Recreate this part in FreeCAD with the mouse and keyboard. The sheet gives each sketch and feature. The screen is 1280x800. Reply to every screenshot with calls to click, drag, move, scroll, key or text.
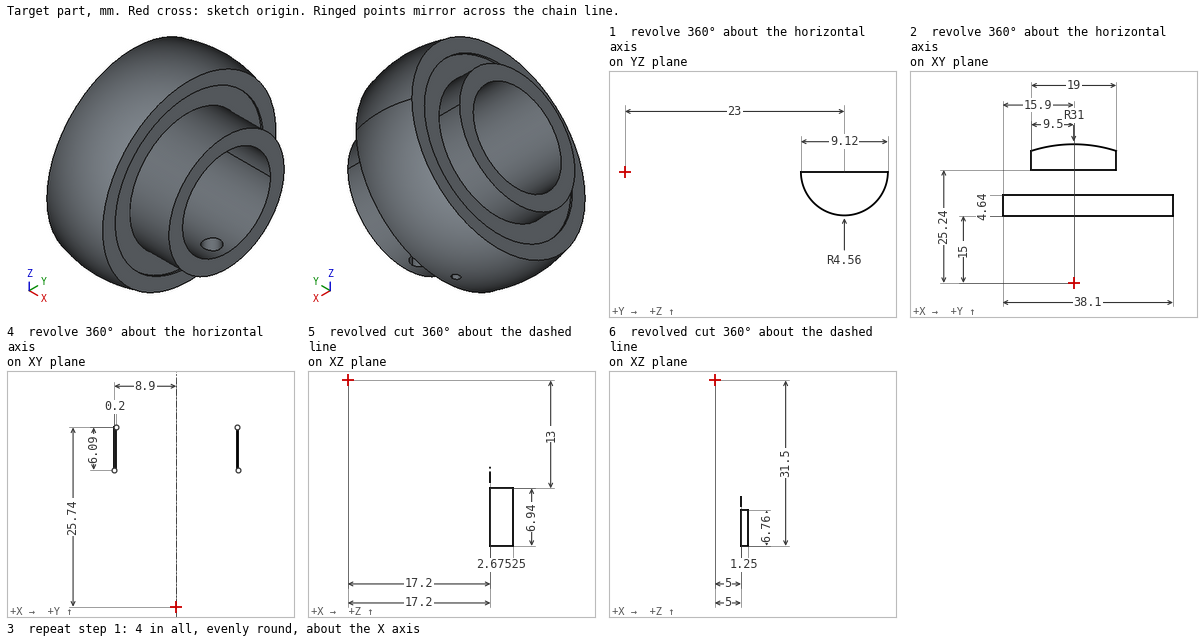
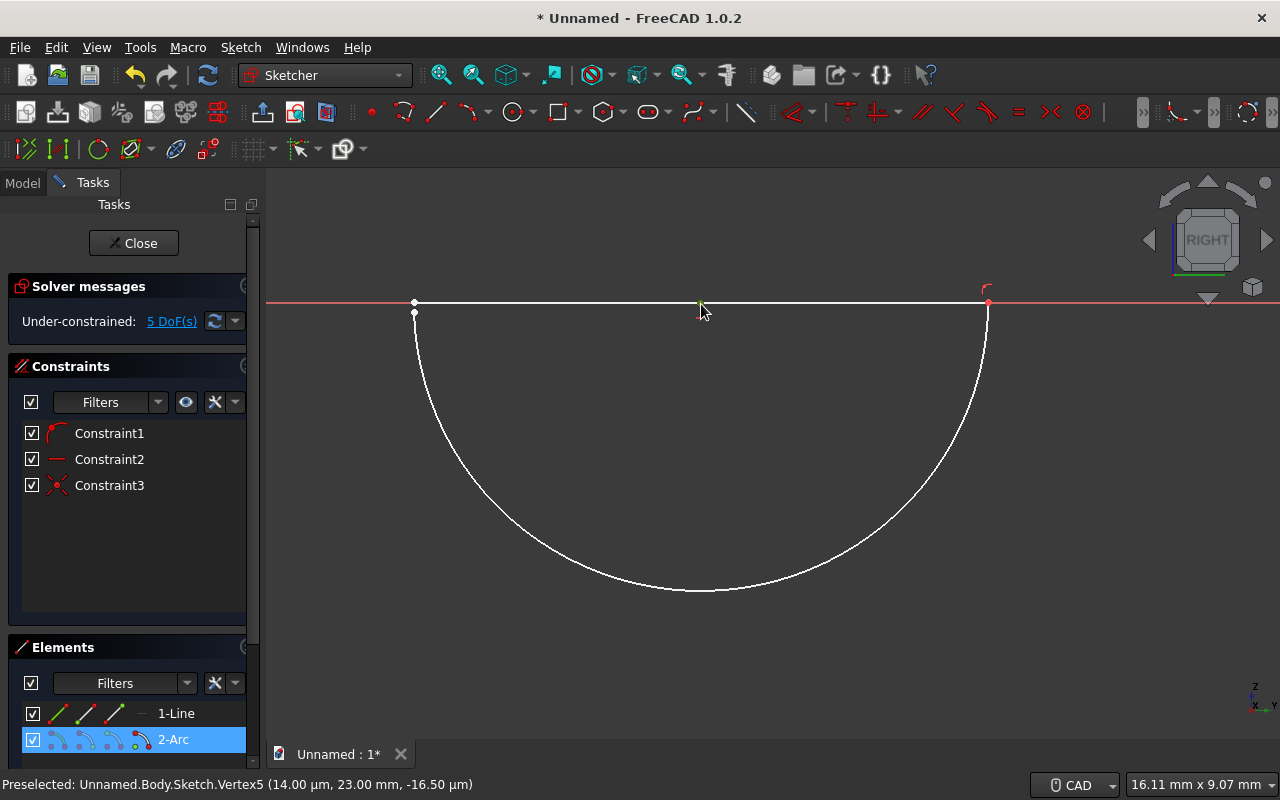
click(353, 303)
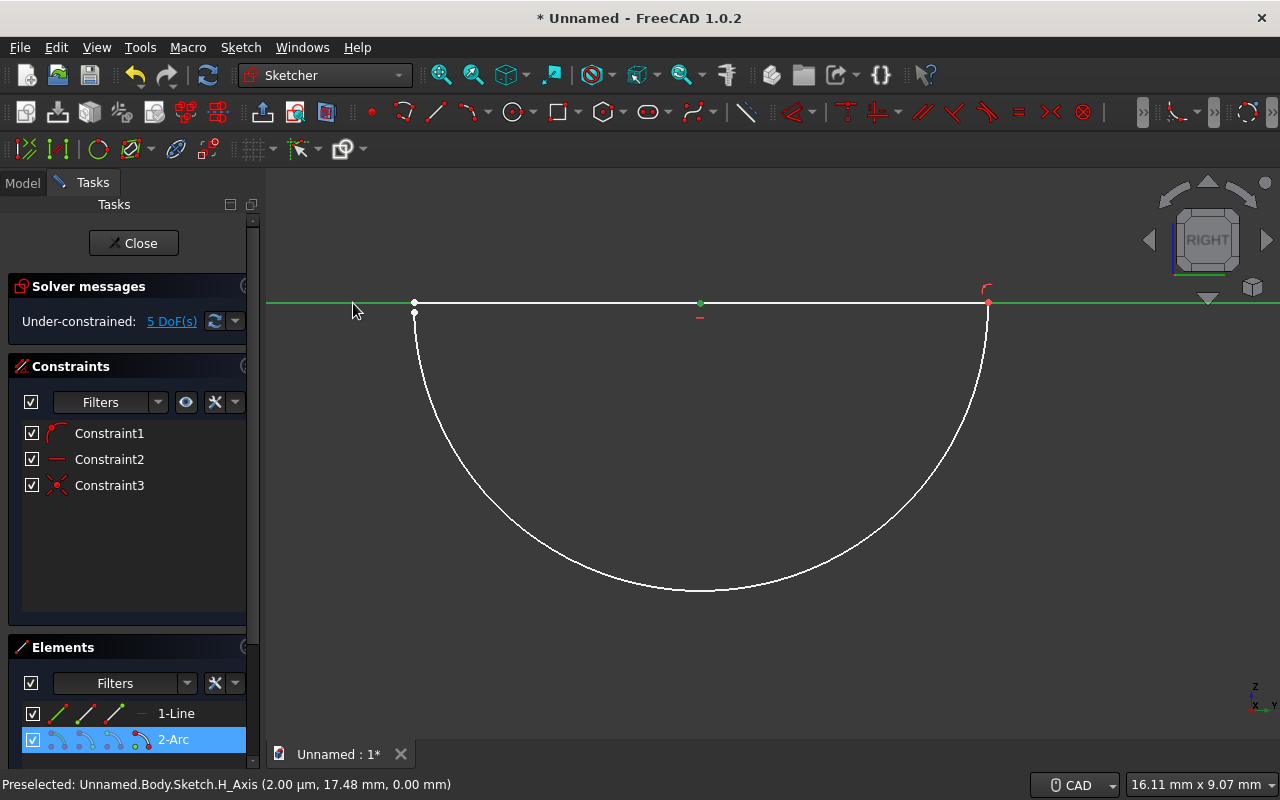
click(846, 112)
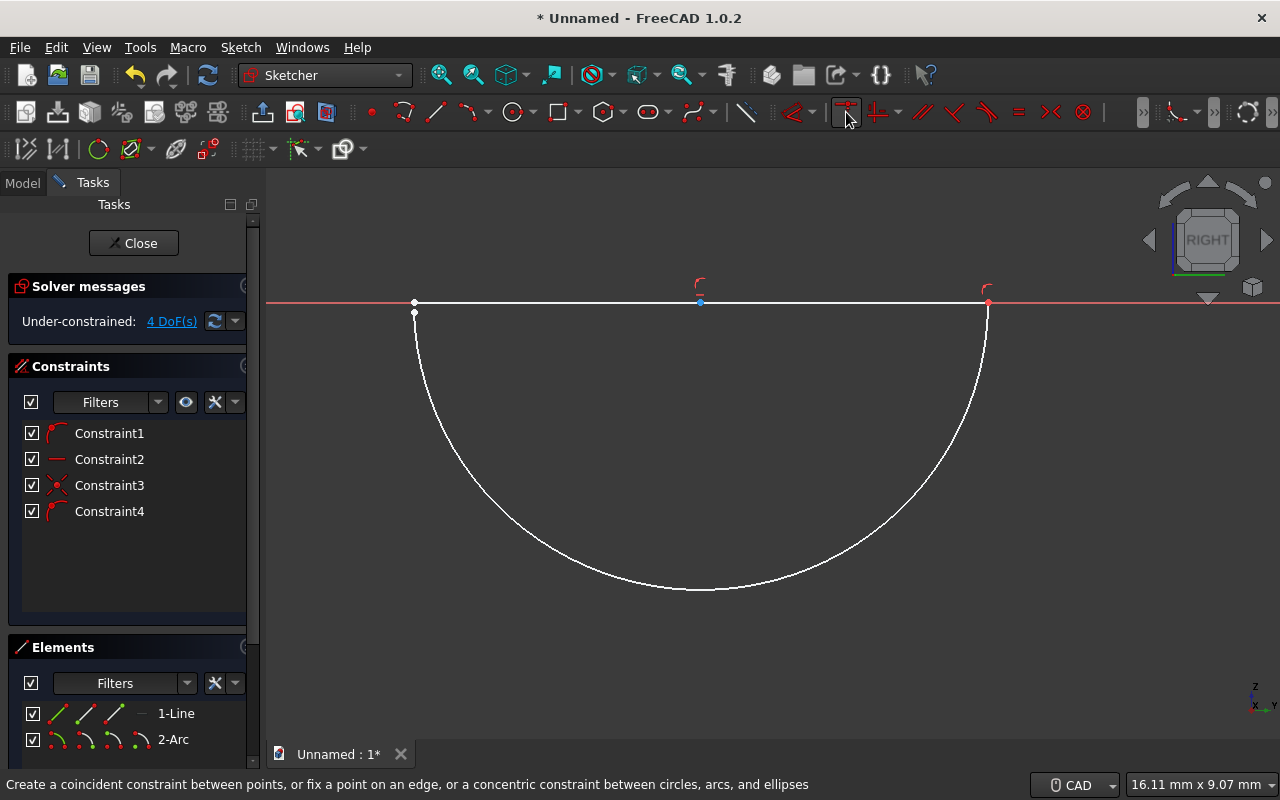
click(792, 112)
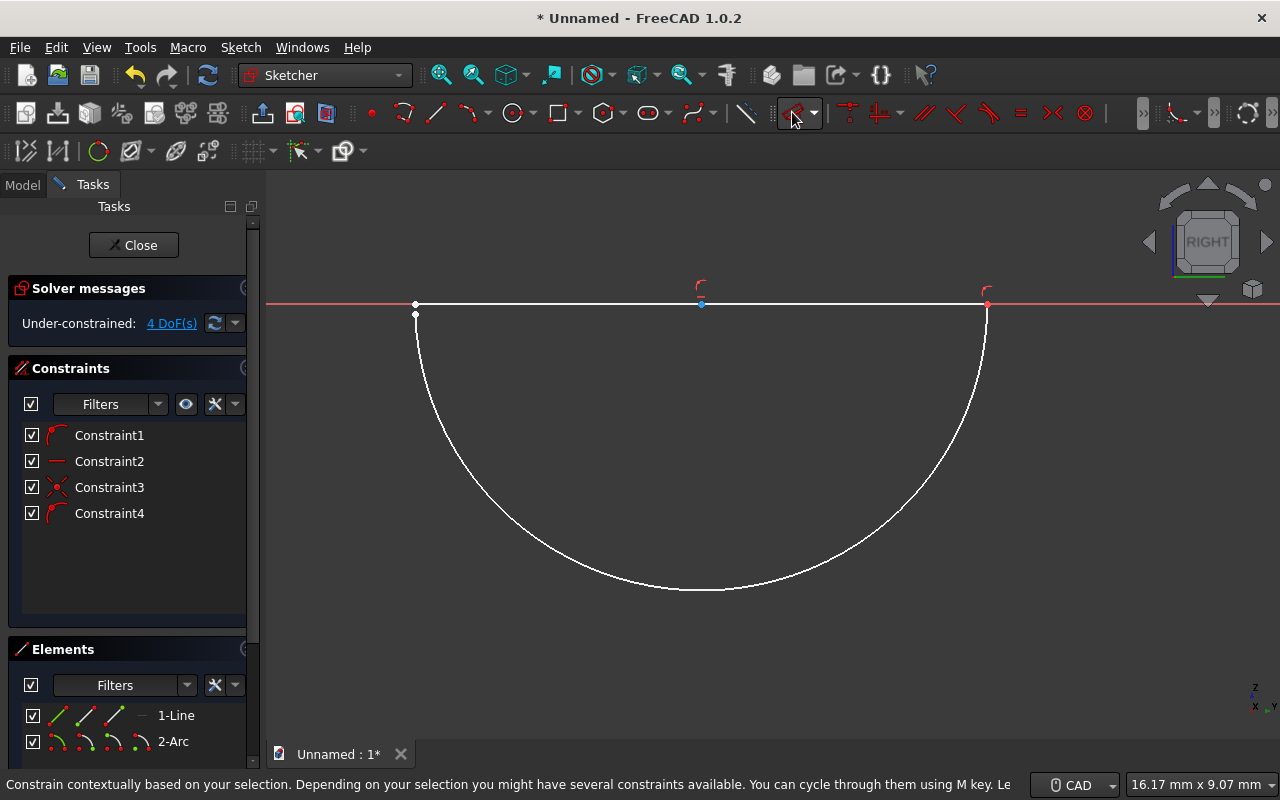
click(539, 540)
click(521, 566)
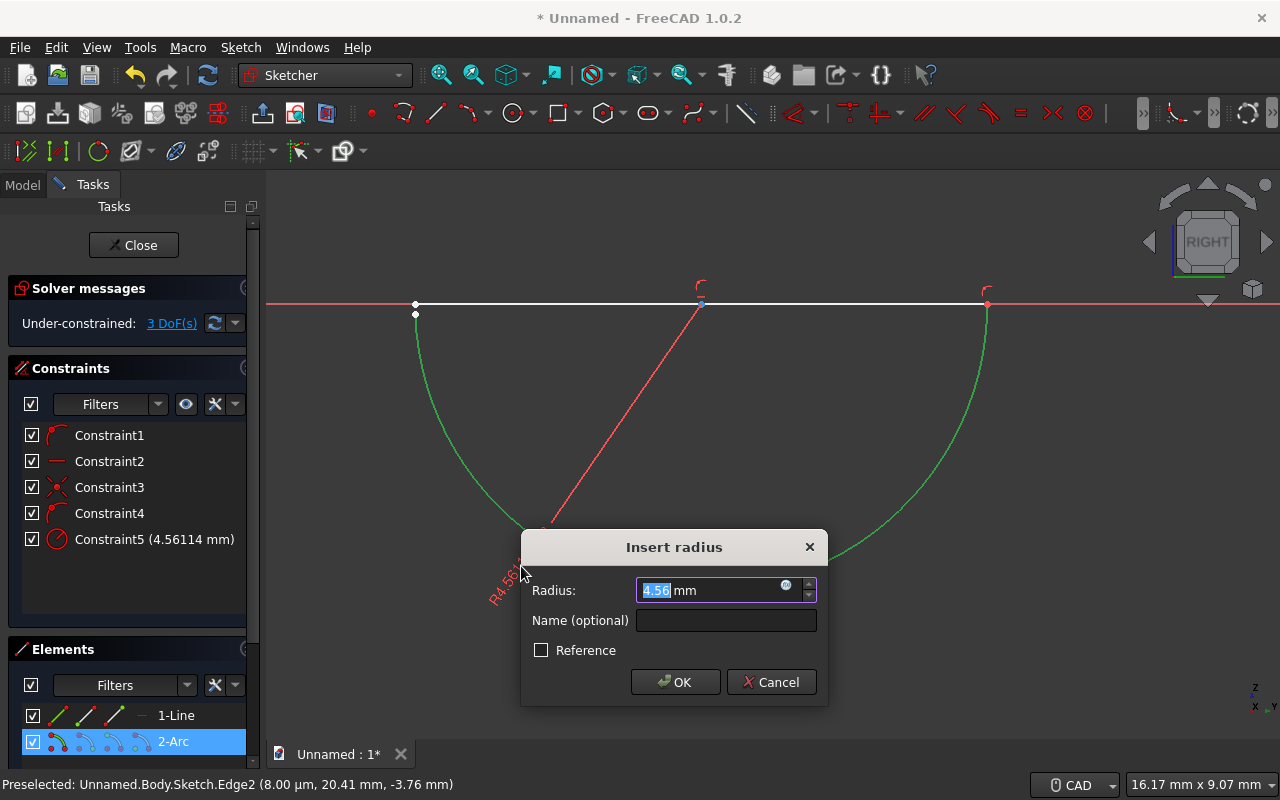
text(4.56)
key(Return)
key(Escape)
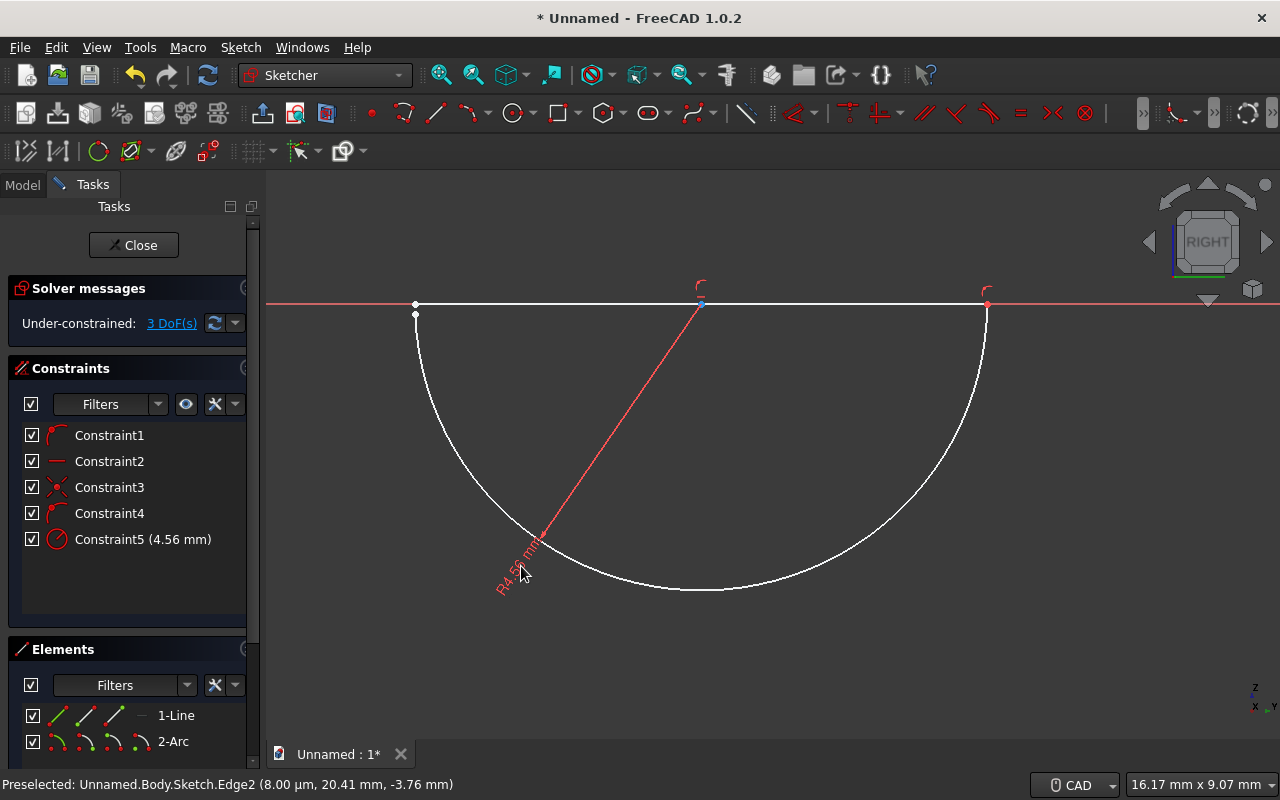
click(415, 314)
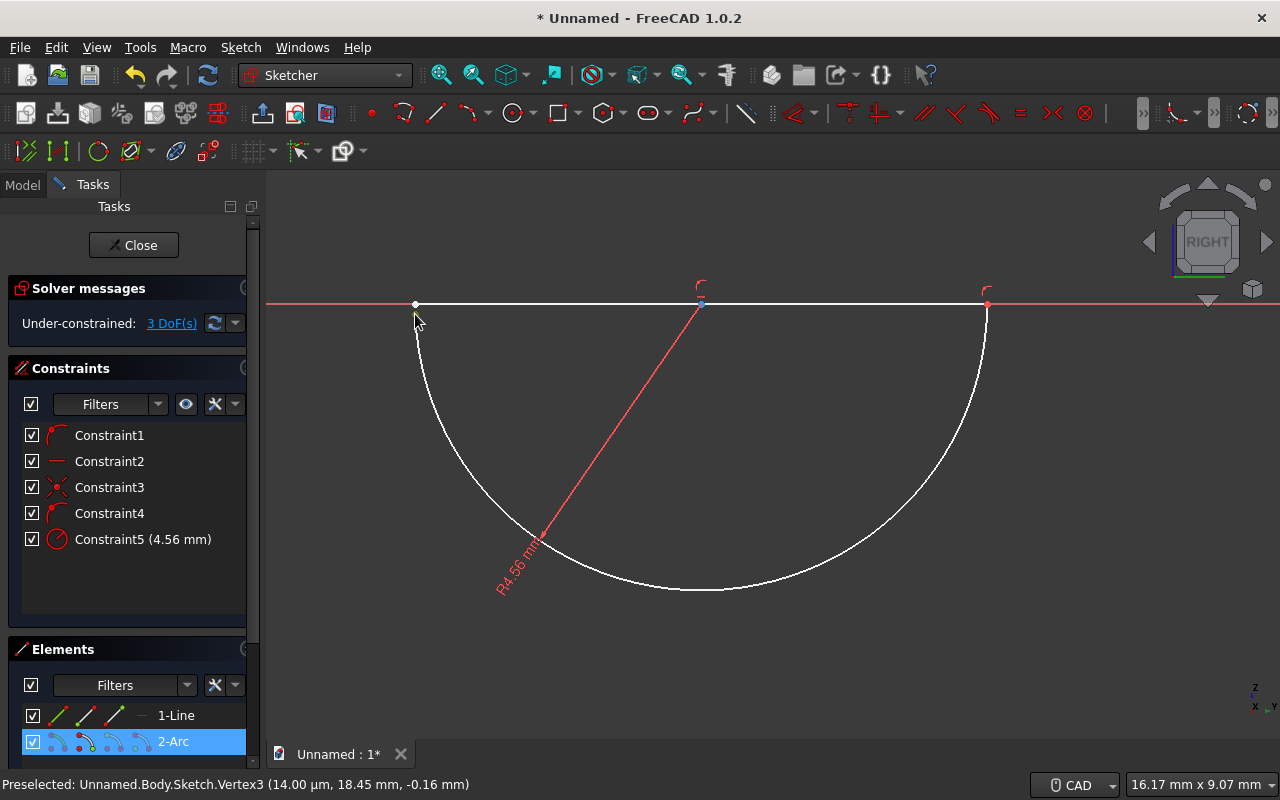
click(353, 304)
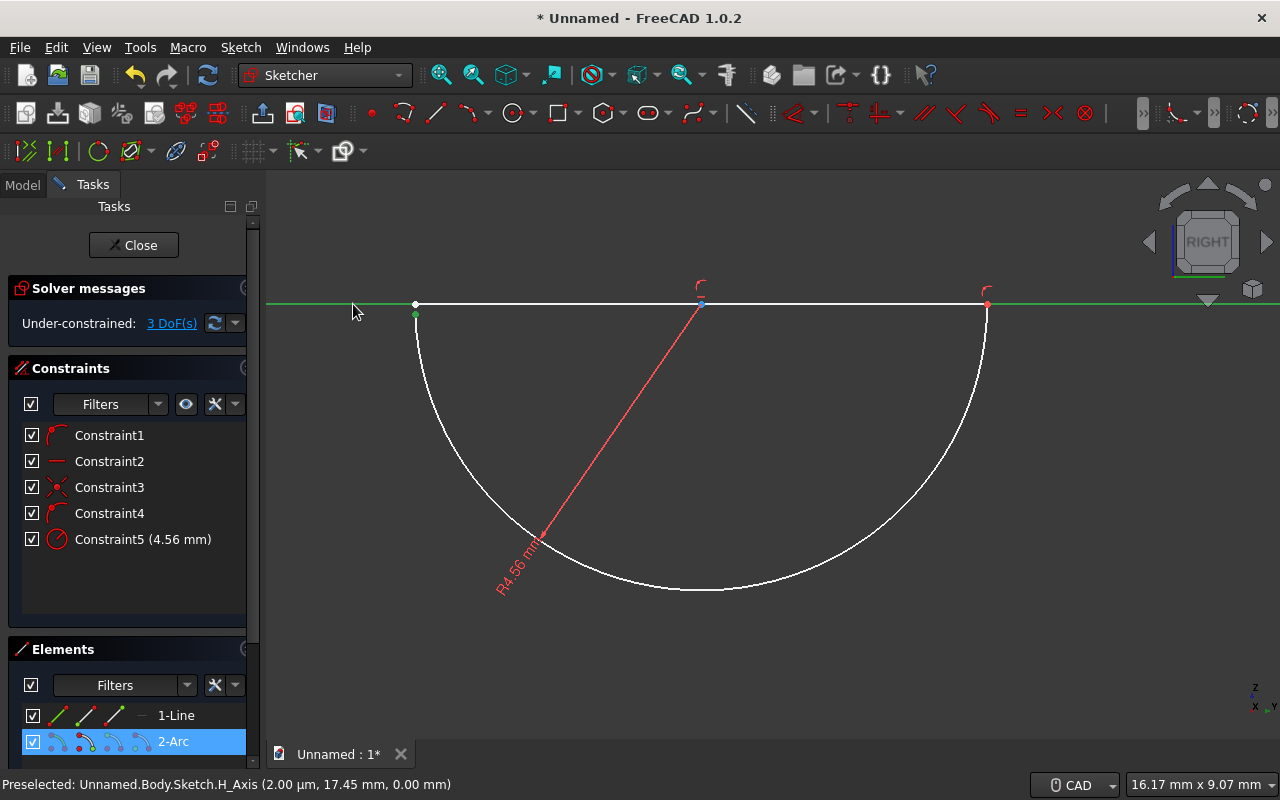
click(848, 114)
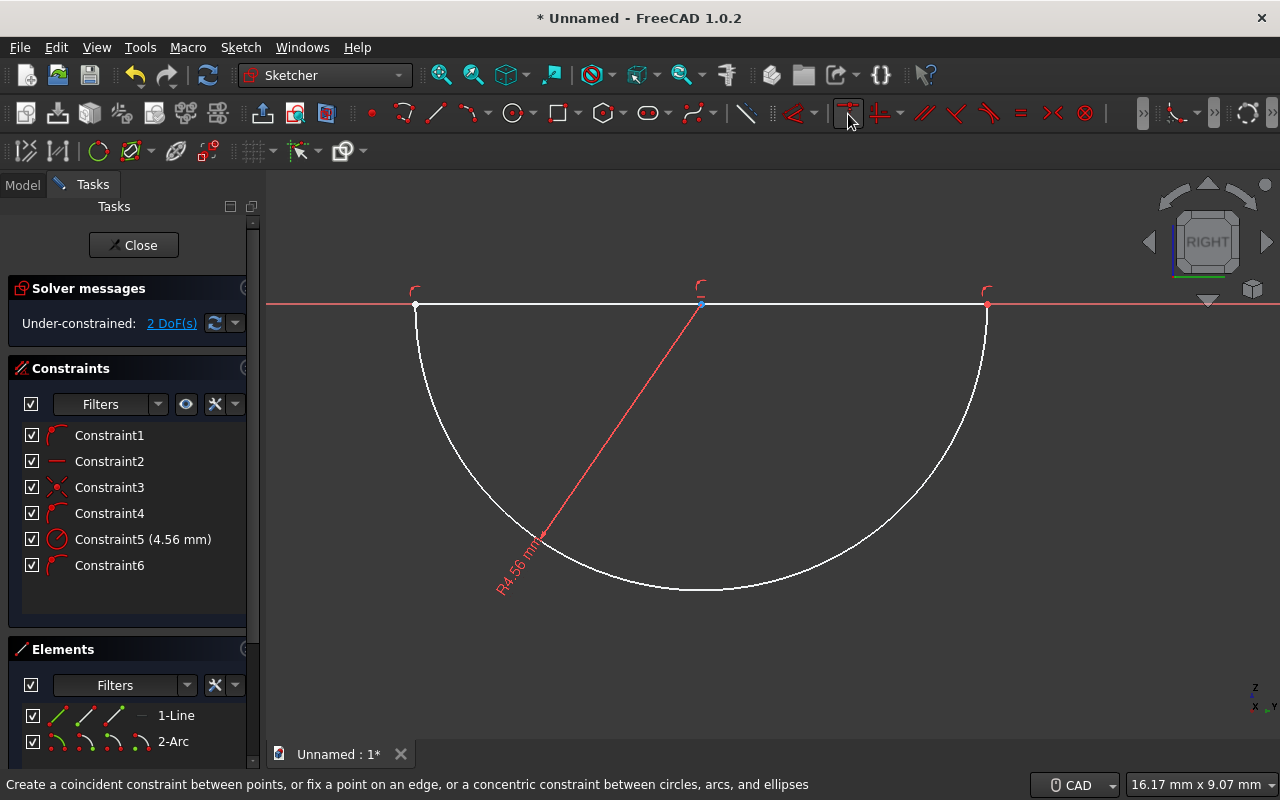
click(794, 114)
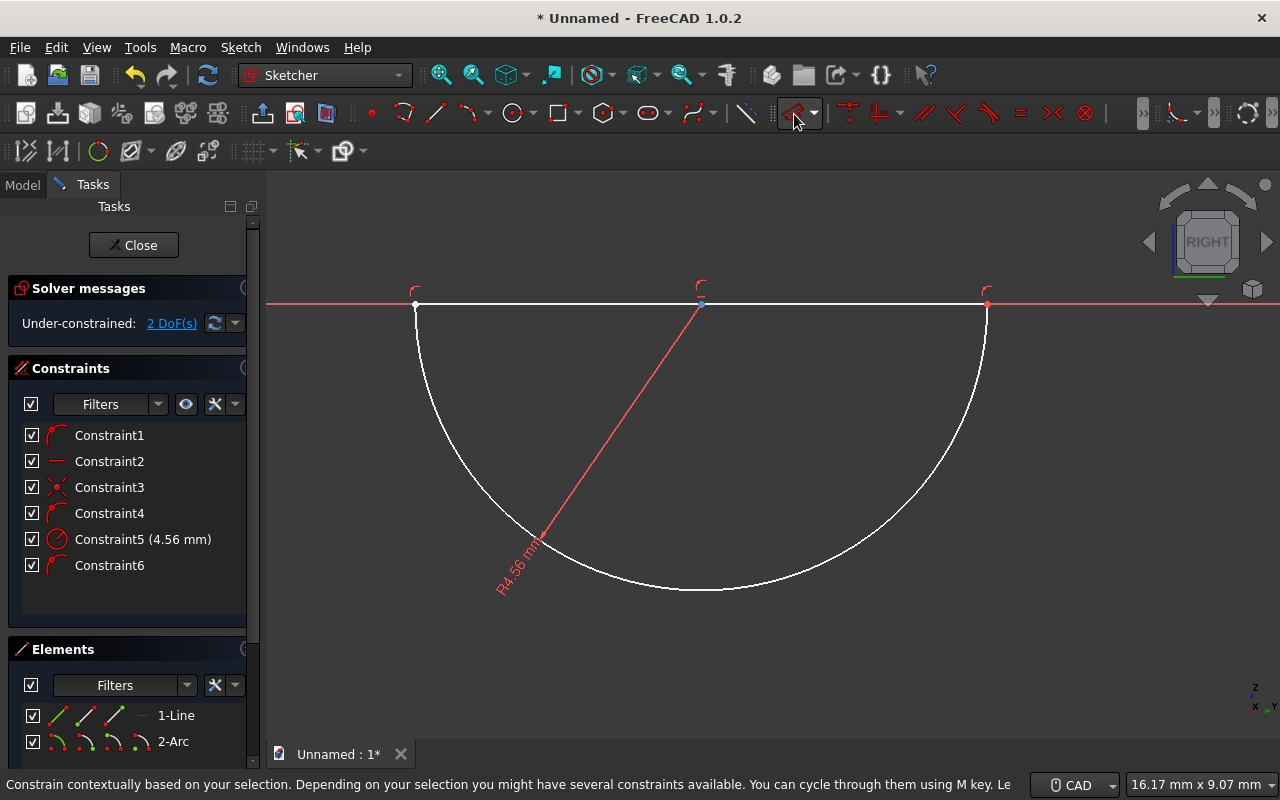
click(701, 304)
click(498, 270)